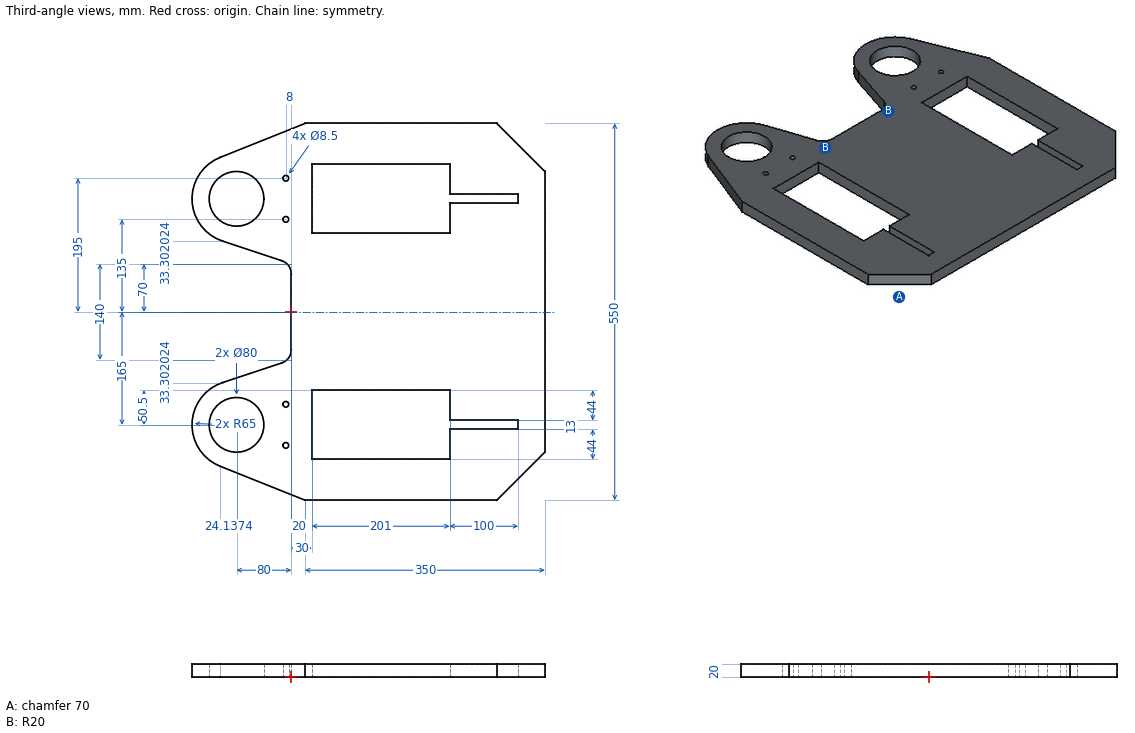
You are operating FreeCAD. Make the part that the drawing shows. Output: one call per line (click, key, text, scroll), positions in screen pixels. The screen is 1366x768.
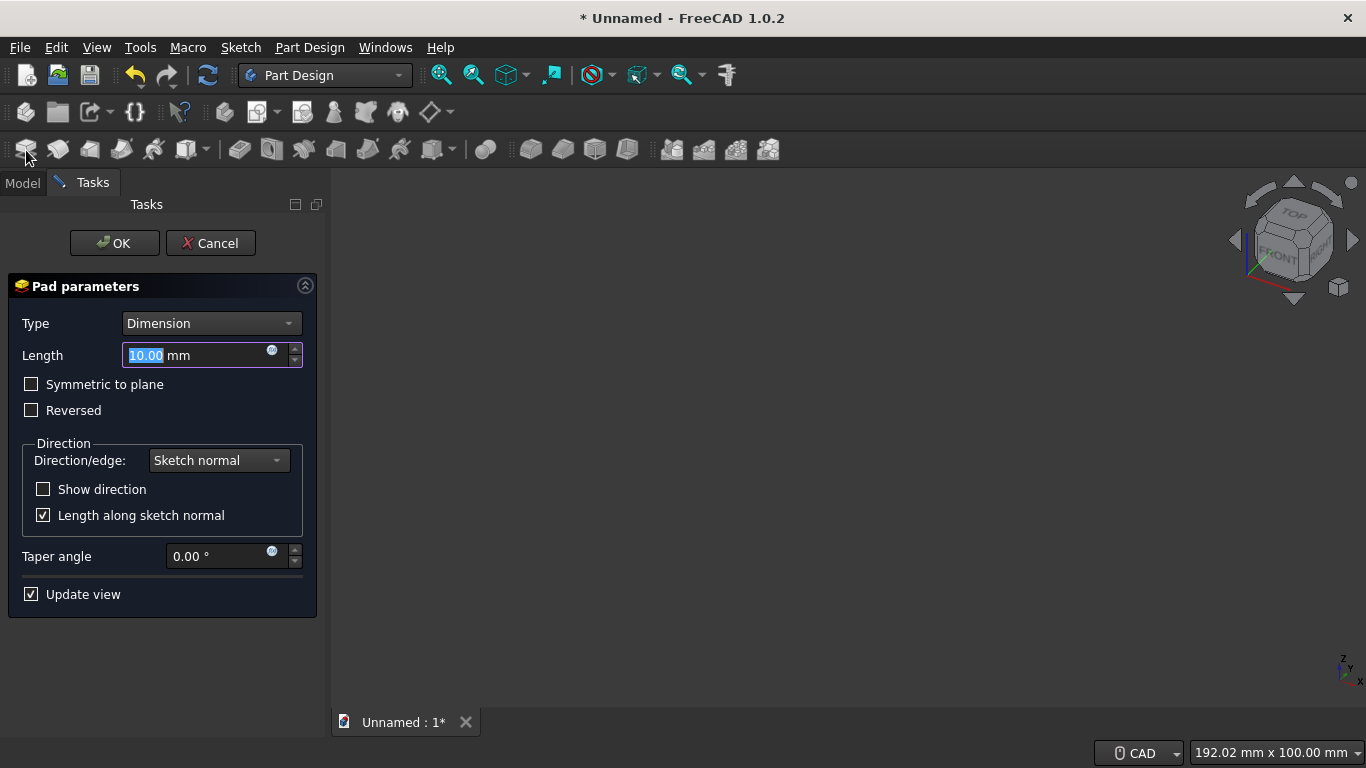
text(20)
key(Tab)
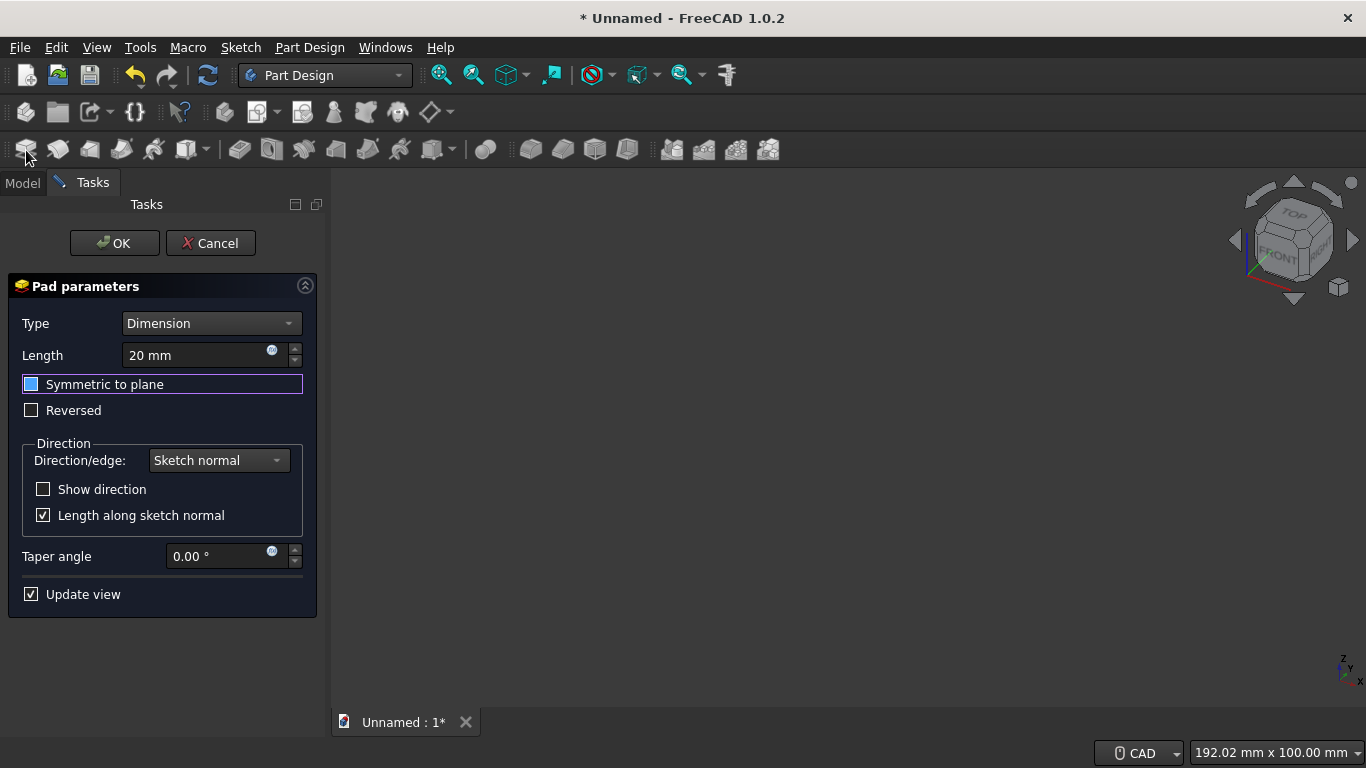
click(115, 243)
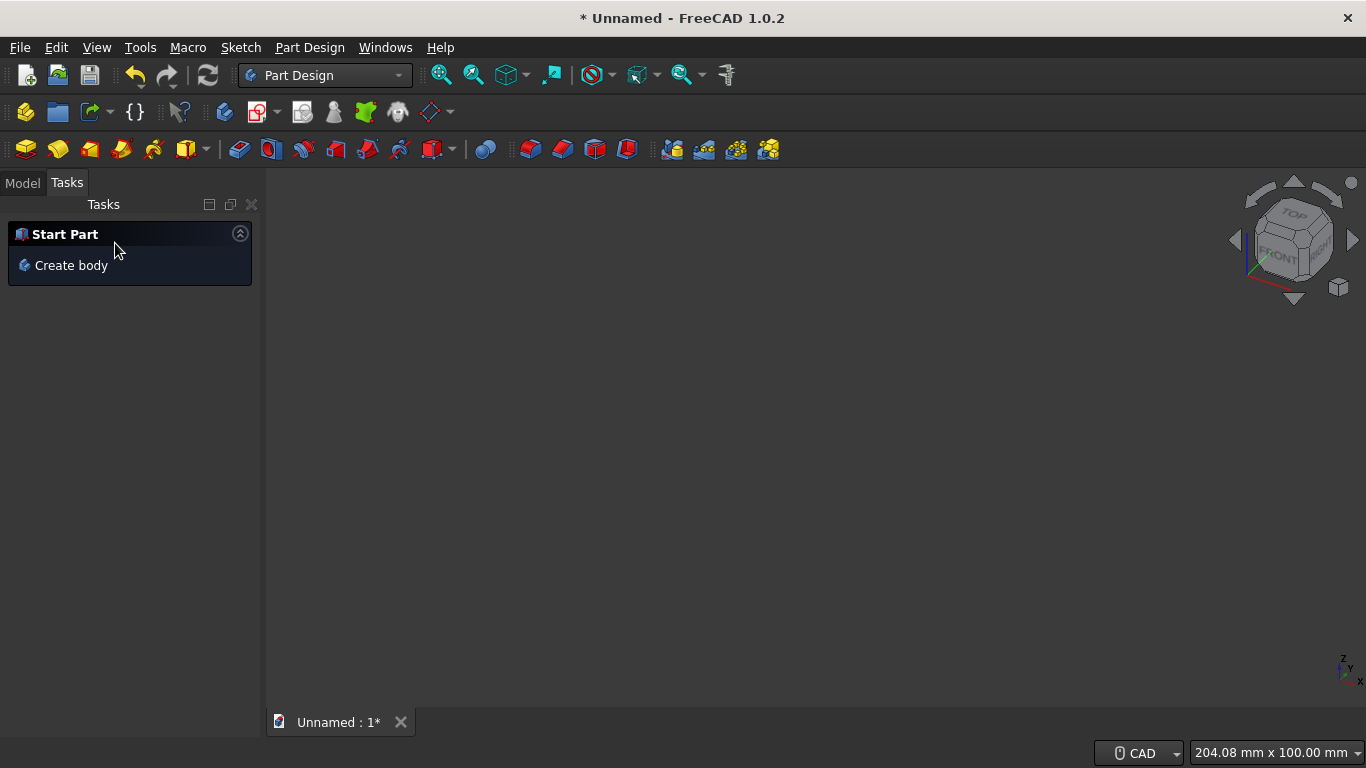
click(442, 76)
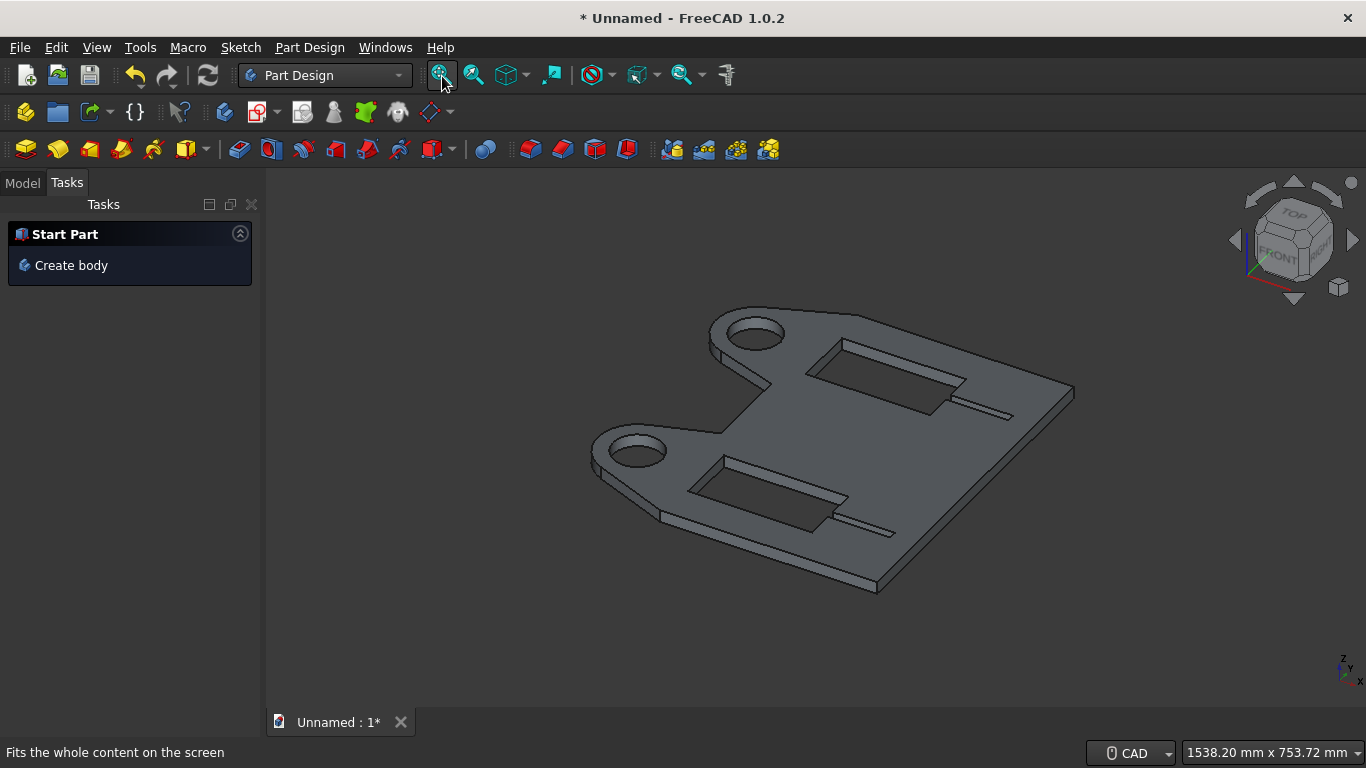
click(862, 446)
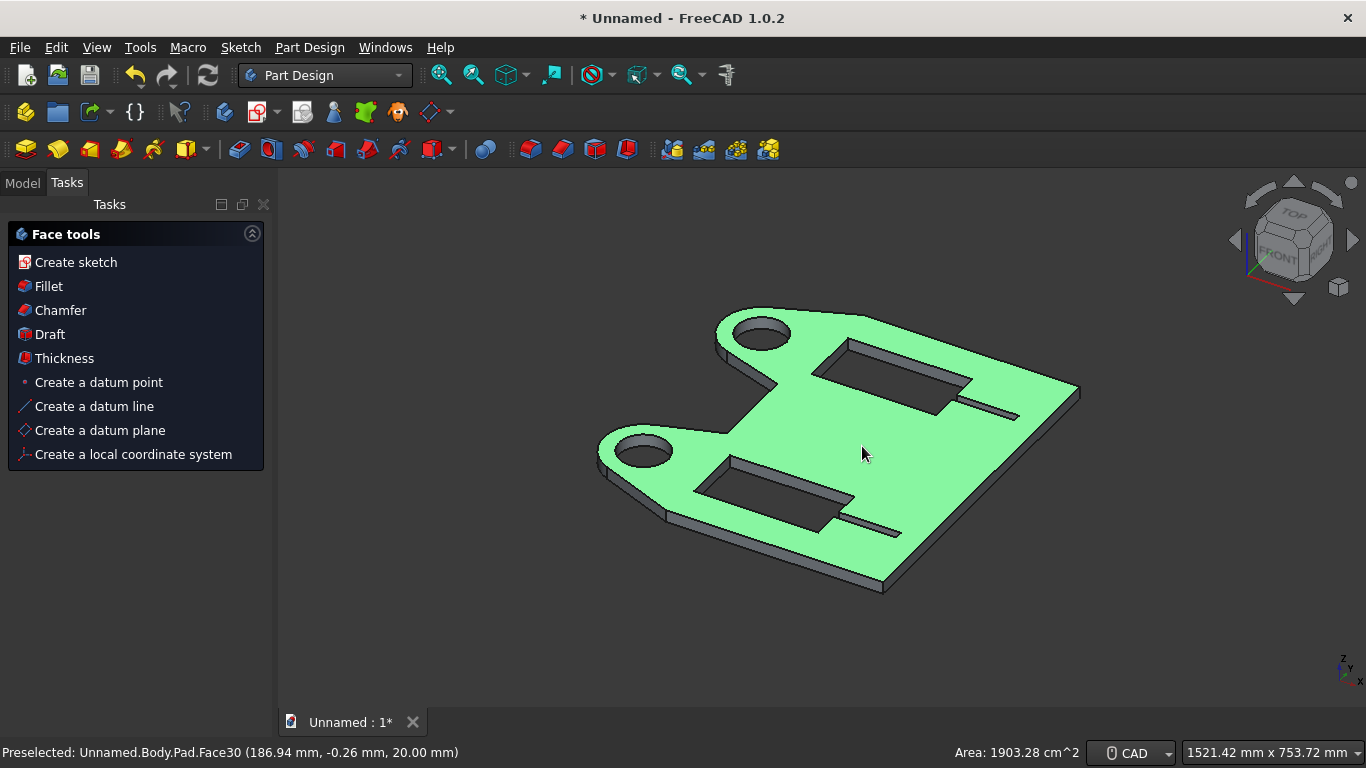
click(258, 112)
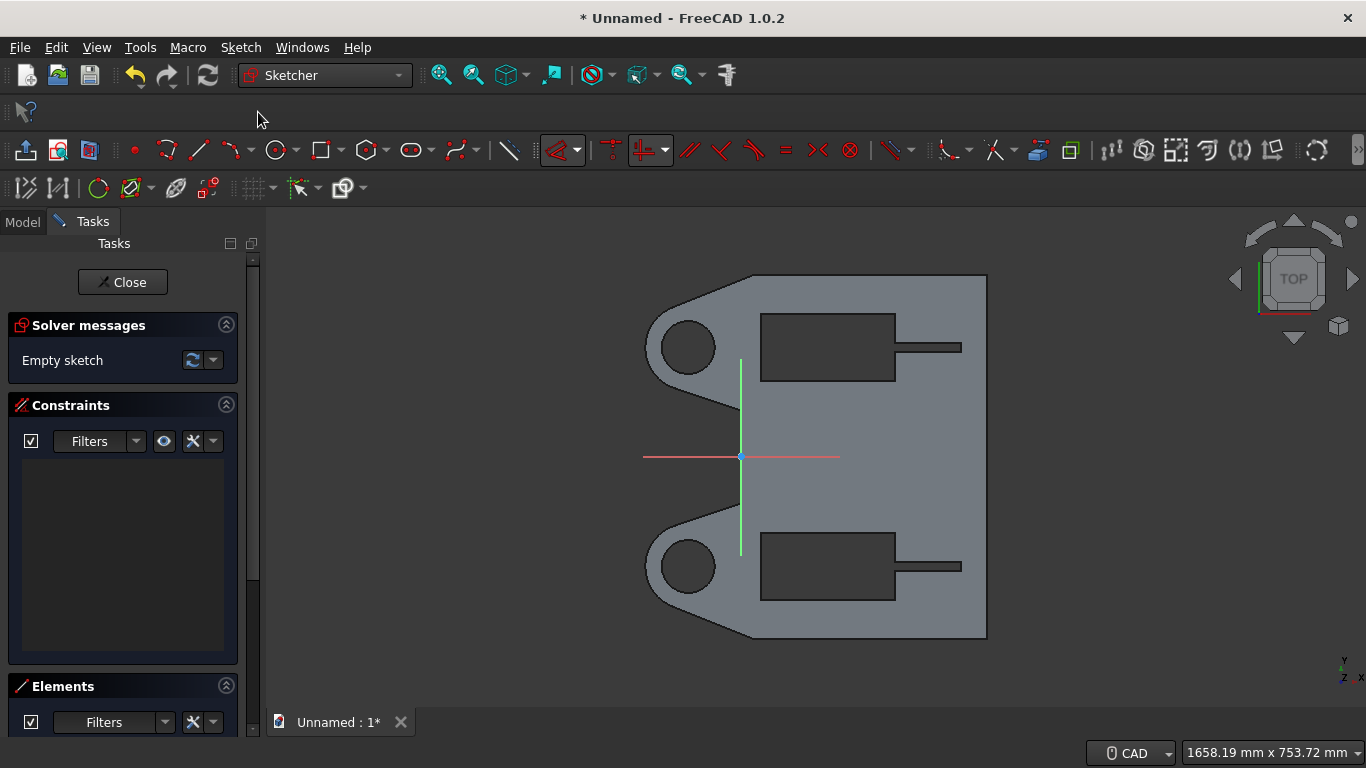
click(276, 150)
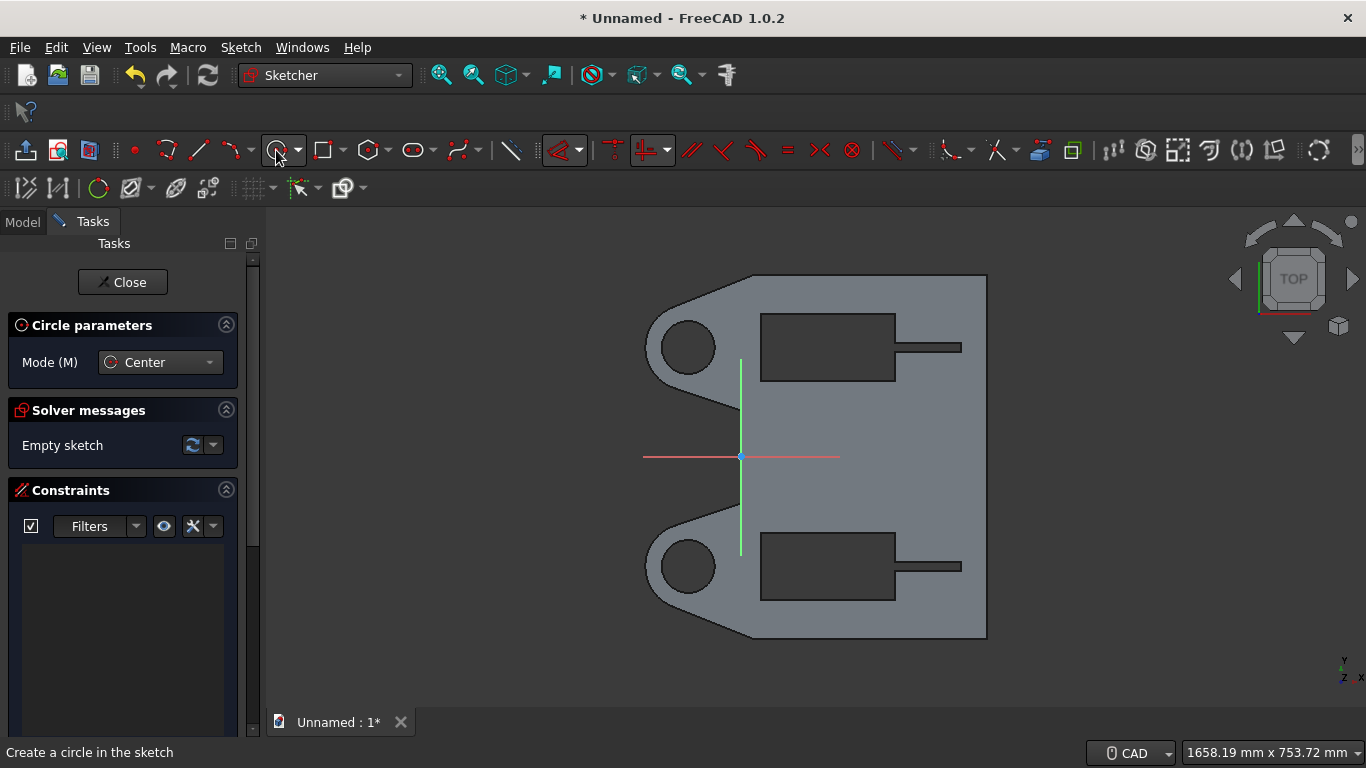
scroll(736, 328, up, 11)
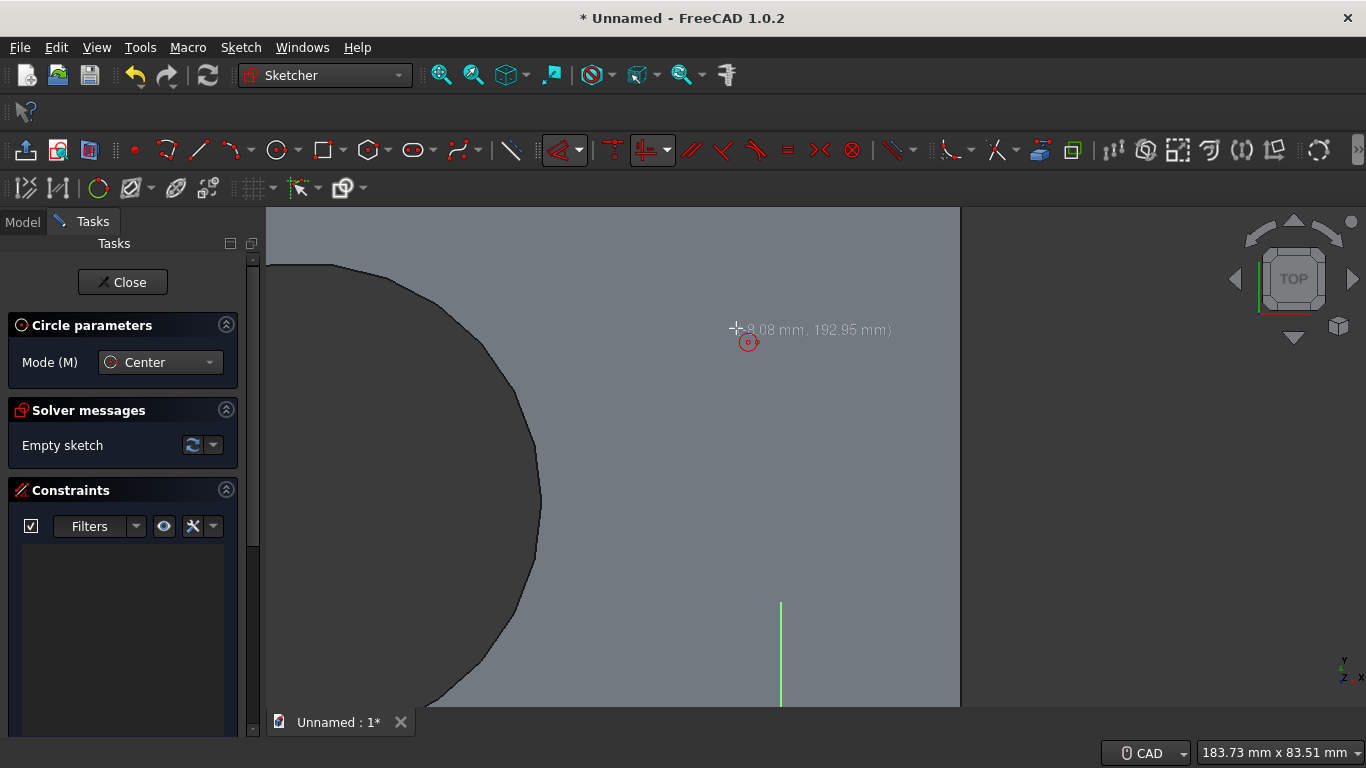
scroll(748, 295, down, 10)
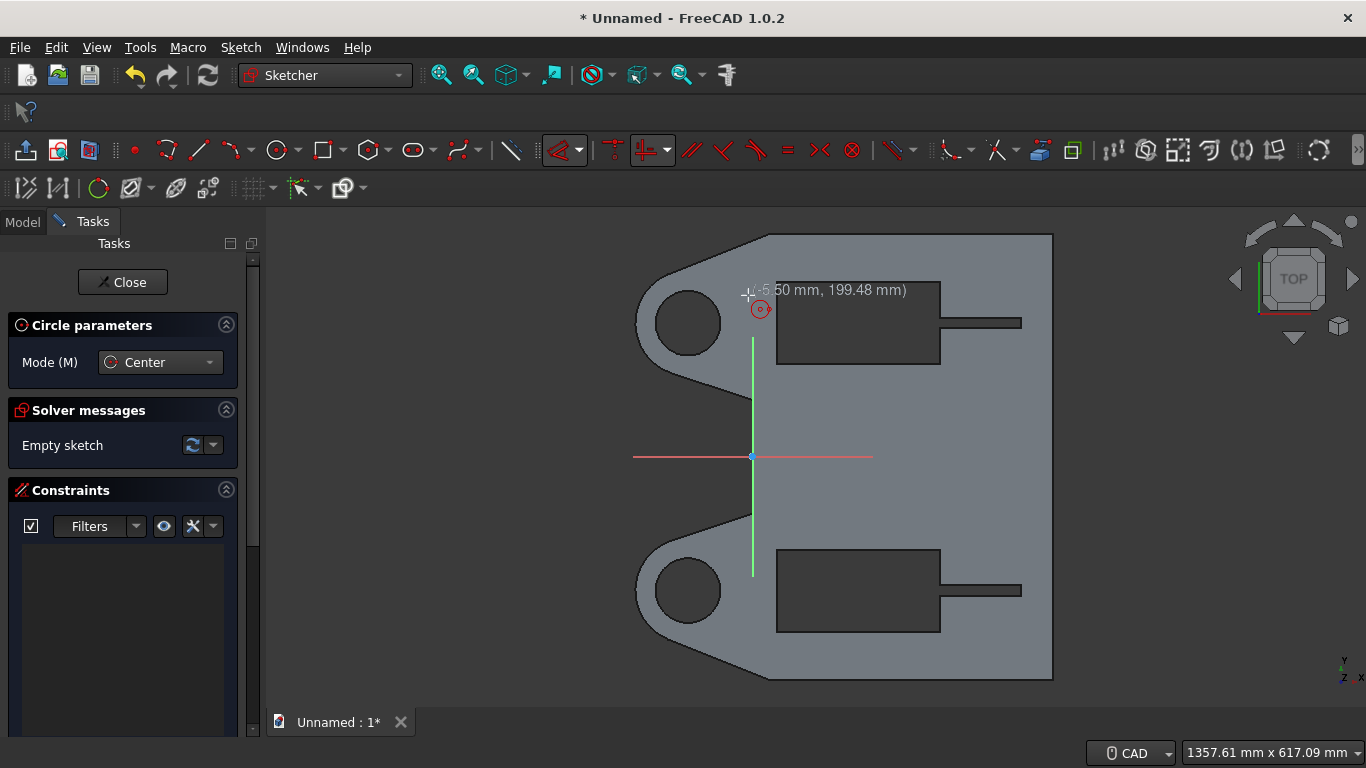
scroll(746, 299, up, 5)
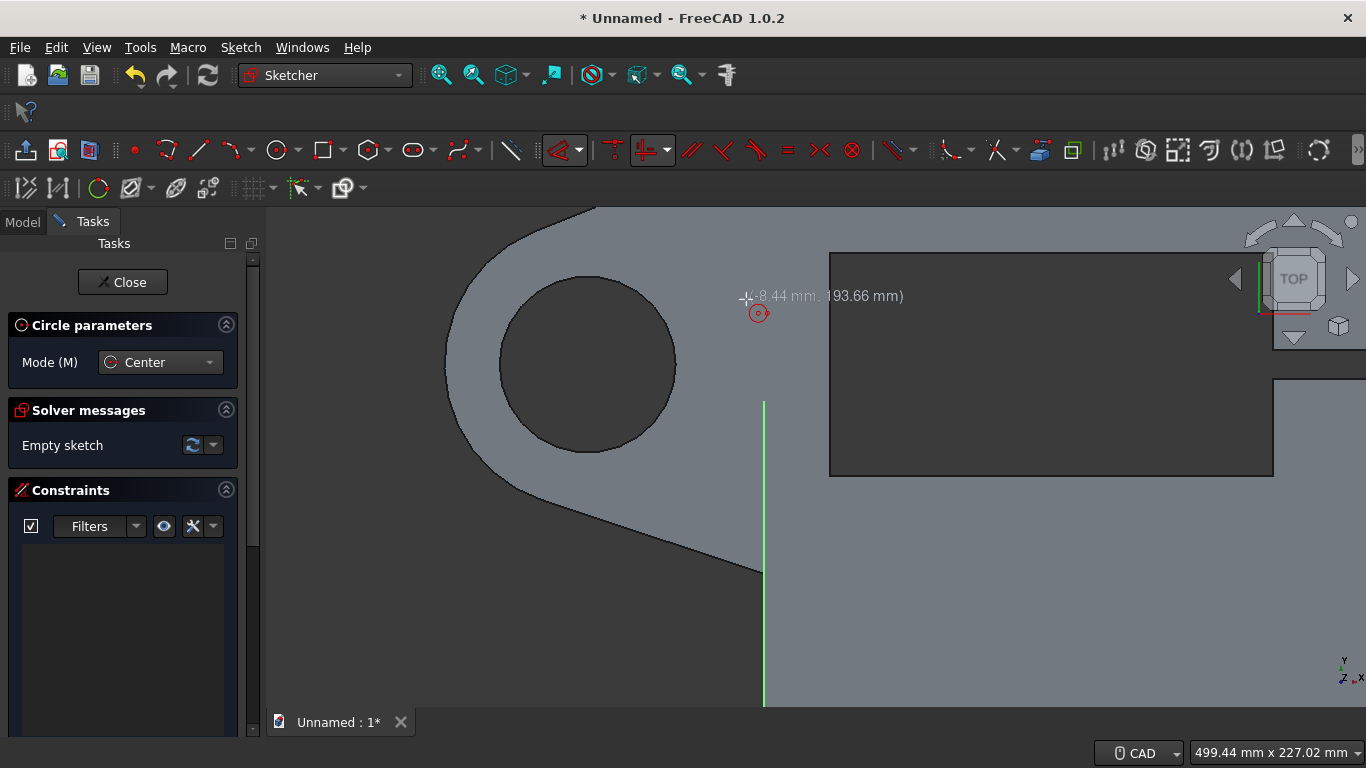
click(746, 298)
move(740, 292)